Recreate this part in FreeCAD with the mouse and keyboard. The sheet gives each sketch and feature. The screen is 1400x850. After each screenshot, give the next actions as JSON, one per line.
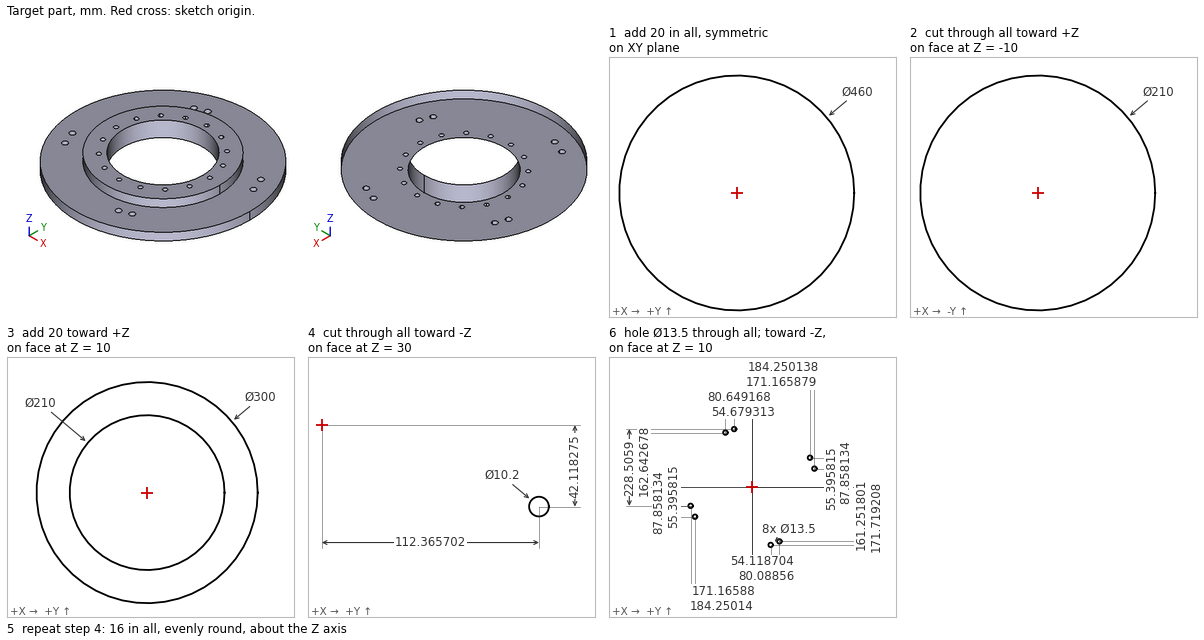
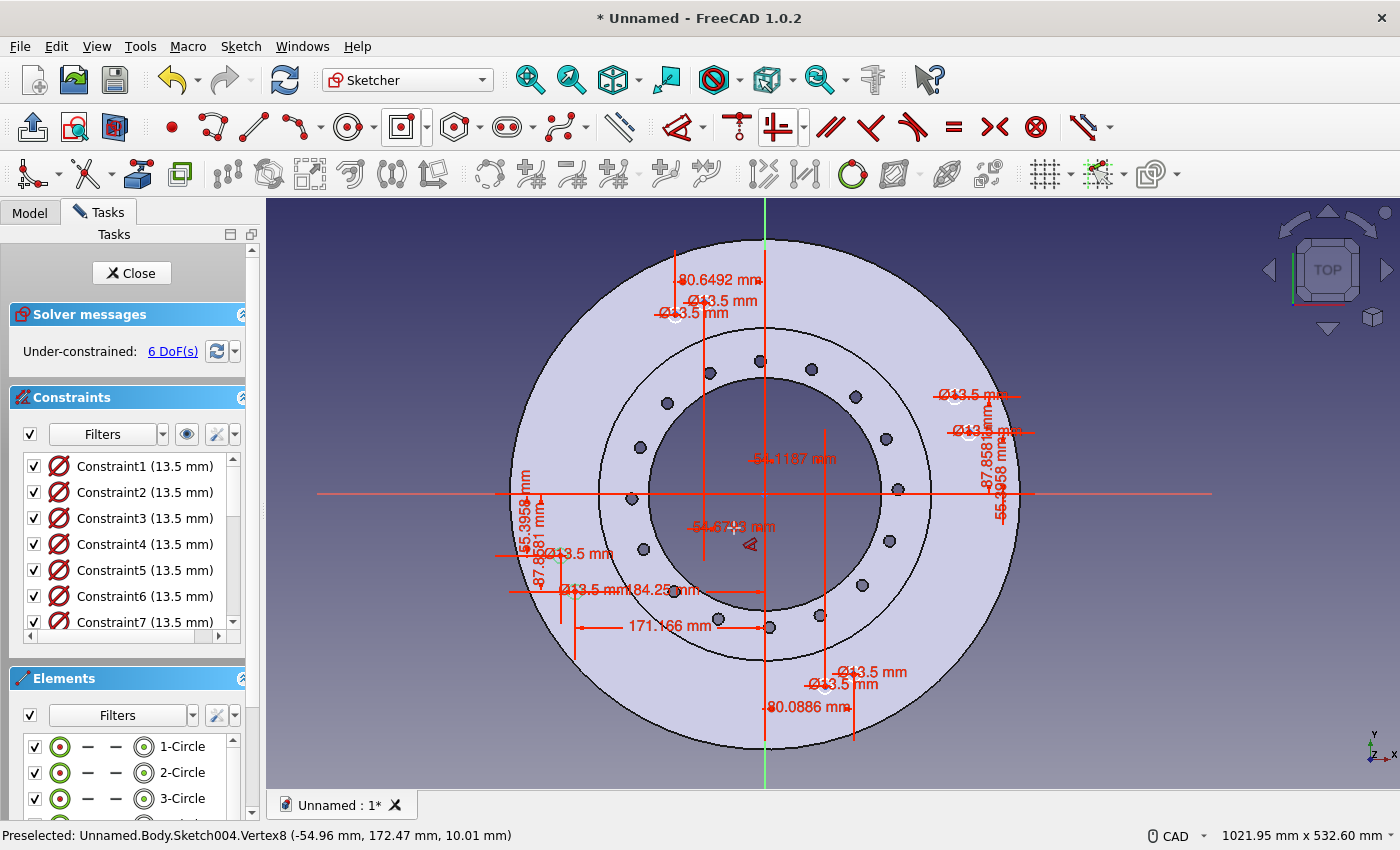
{"action": "left_click", "coordinate": [561, 556]}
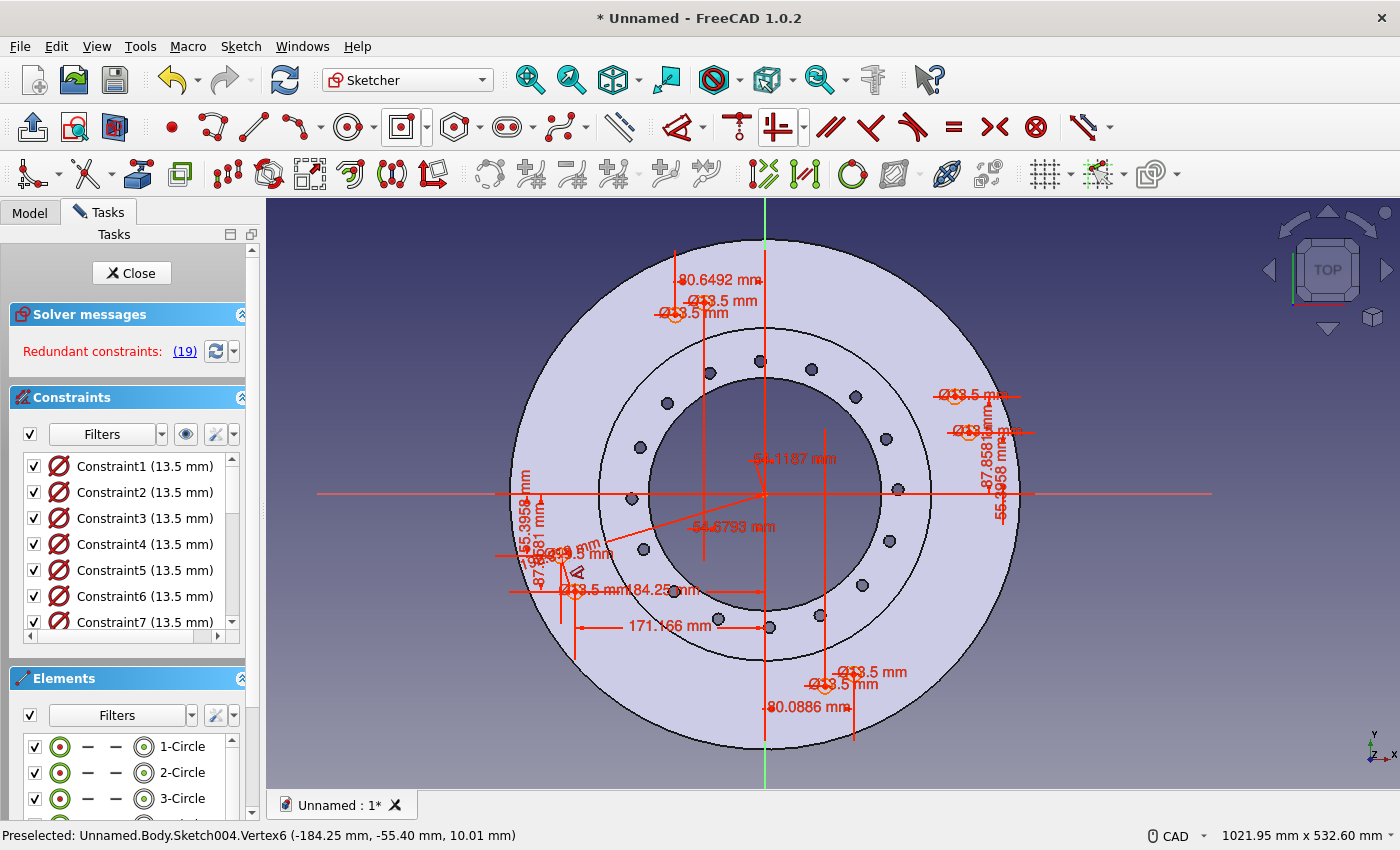
{"action": "left_click", "coordinate": [704, 303]}
{"action": "left_click", "coordinate": [527, 429]}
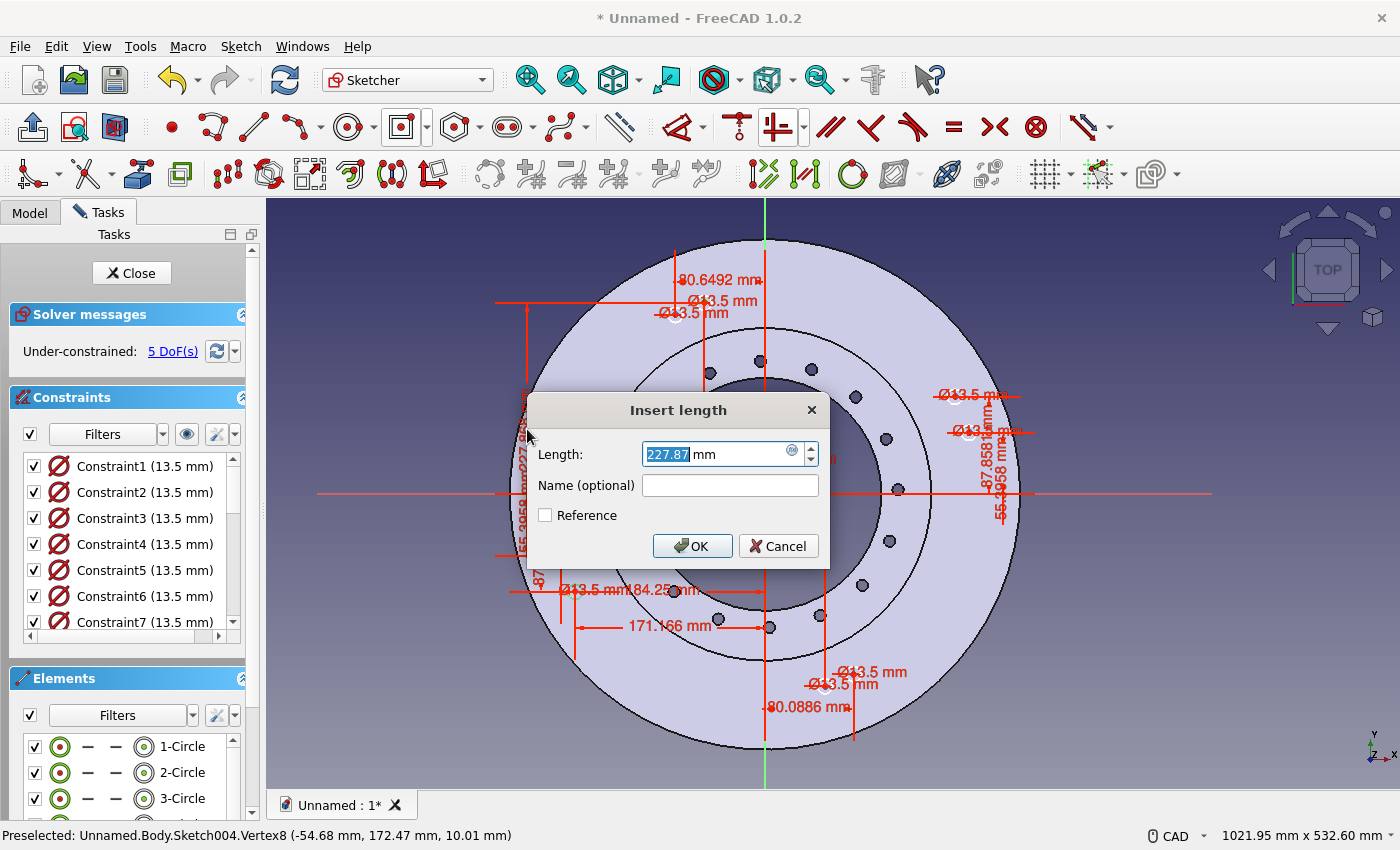
{"action": "type", "text": "228.5059"}
{"action": "key", "text": "Return"}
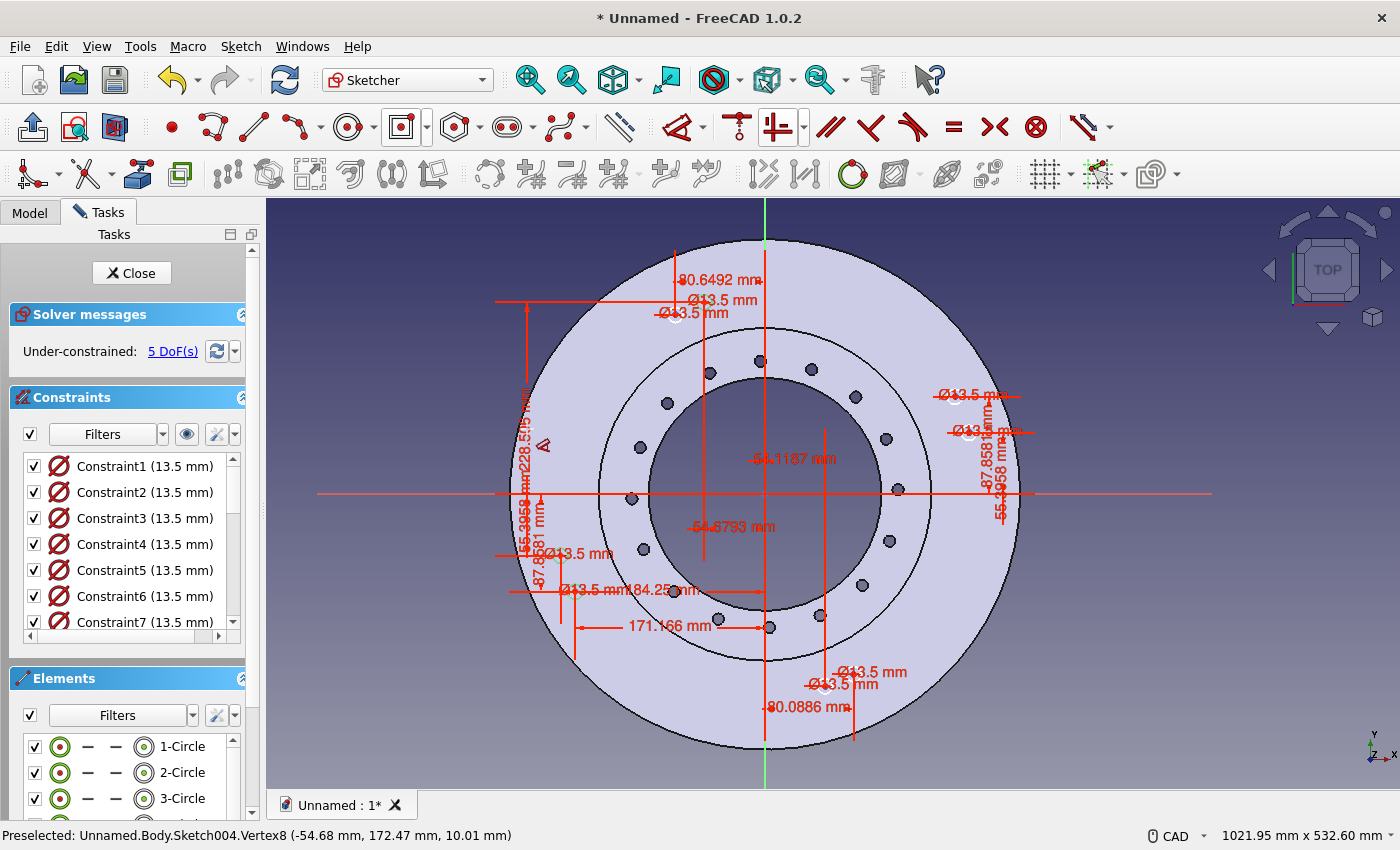
{"action": "left_click", "coordinate": [825, 686]}
{"action": "left_click", "coordinate": [859, 590]}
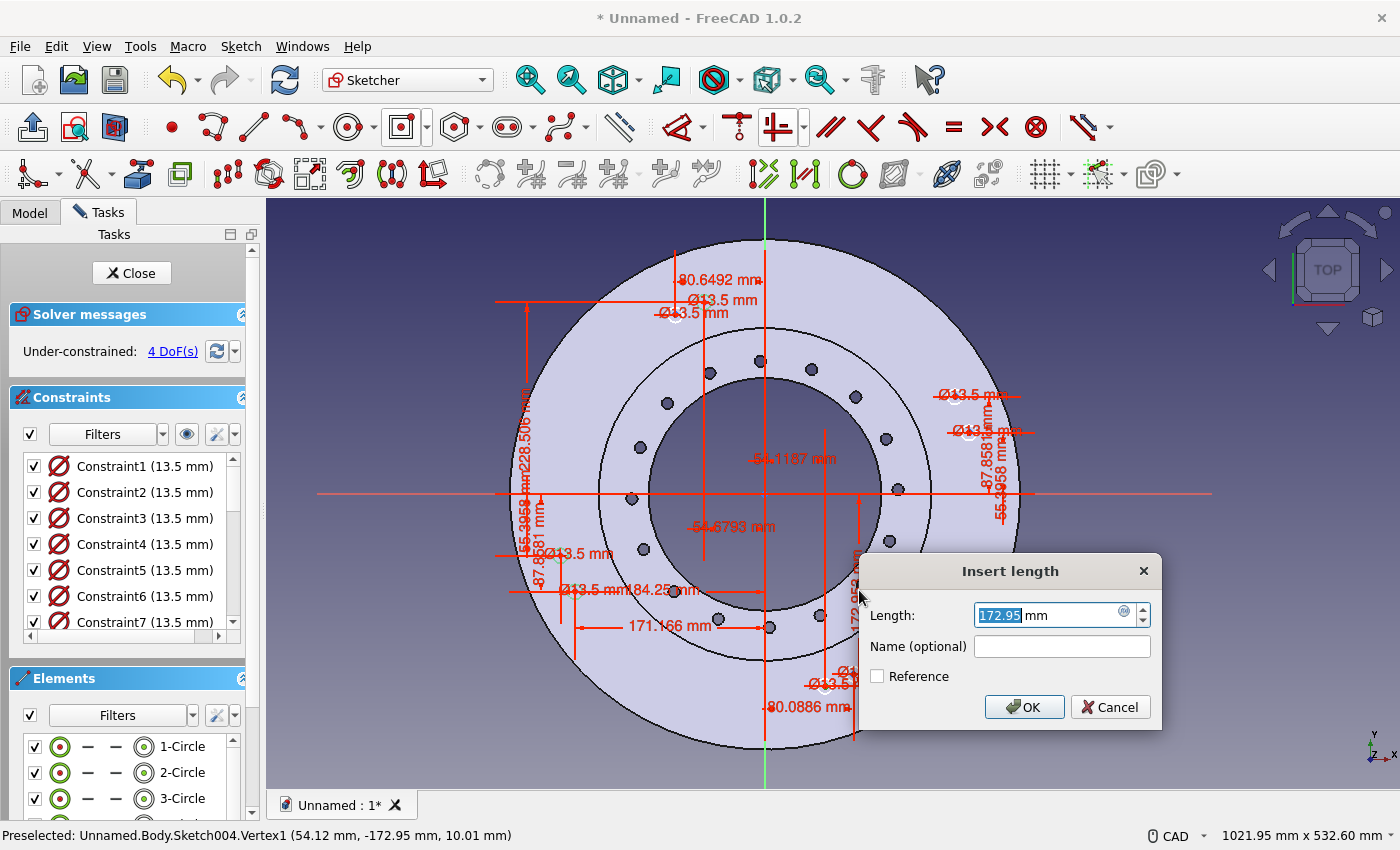
{"action": "type", "text": "171.719208"}
{"action": "key", "text": "Return"}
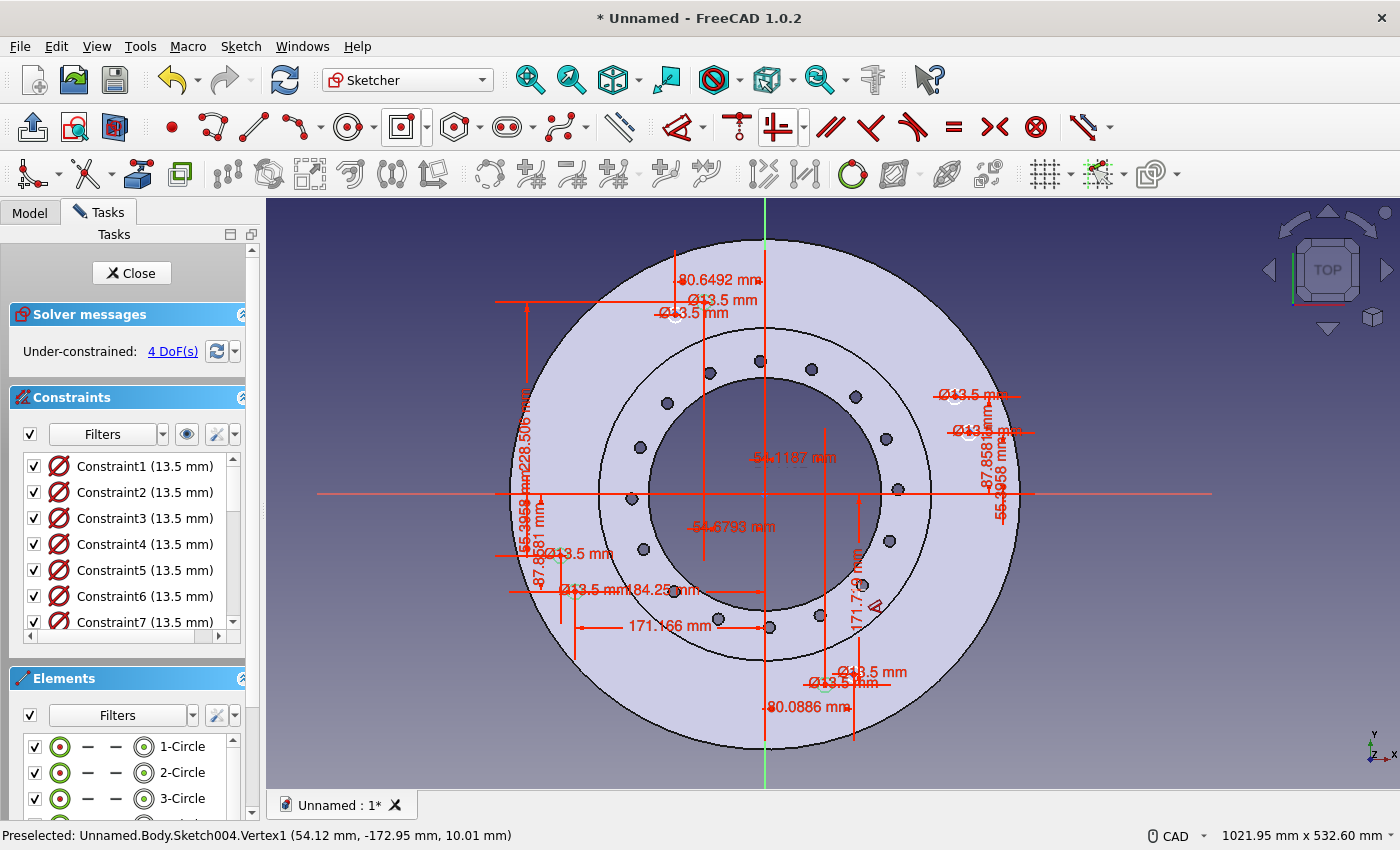
{"action": "left_click", "coordinate": [854, 674]}
{"action": "left_click", "coordinate": [888, 543]}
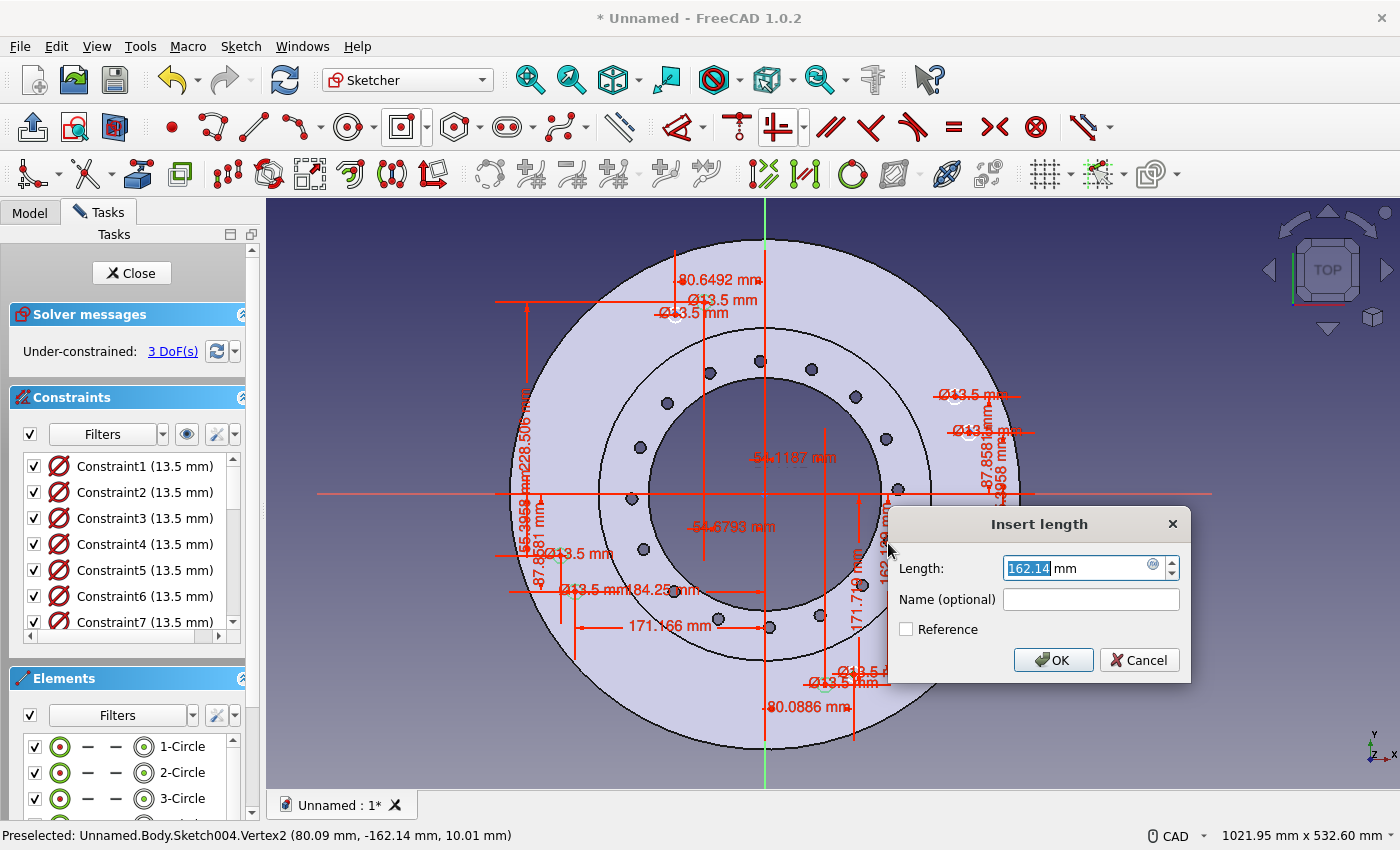
{"action": "type", "text": "161.251801"}
{"action": "key", "text": "Return"}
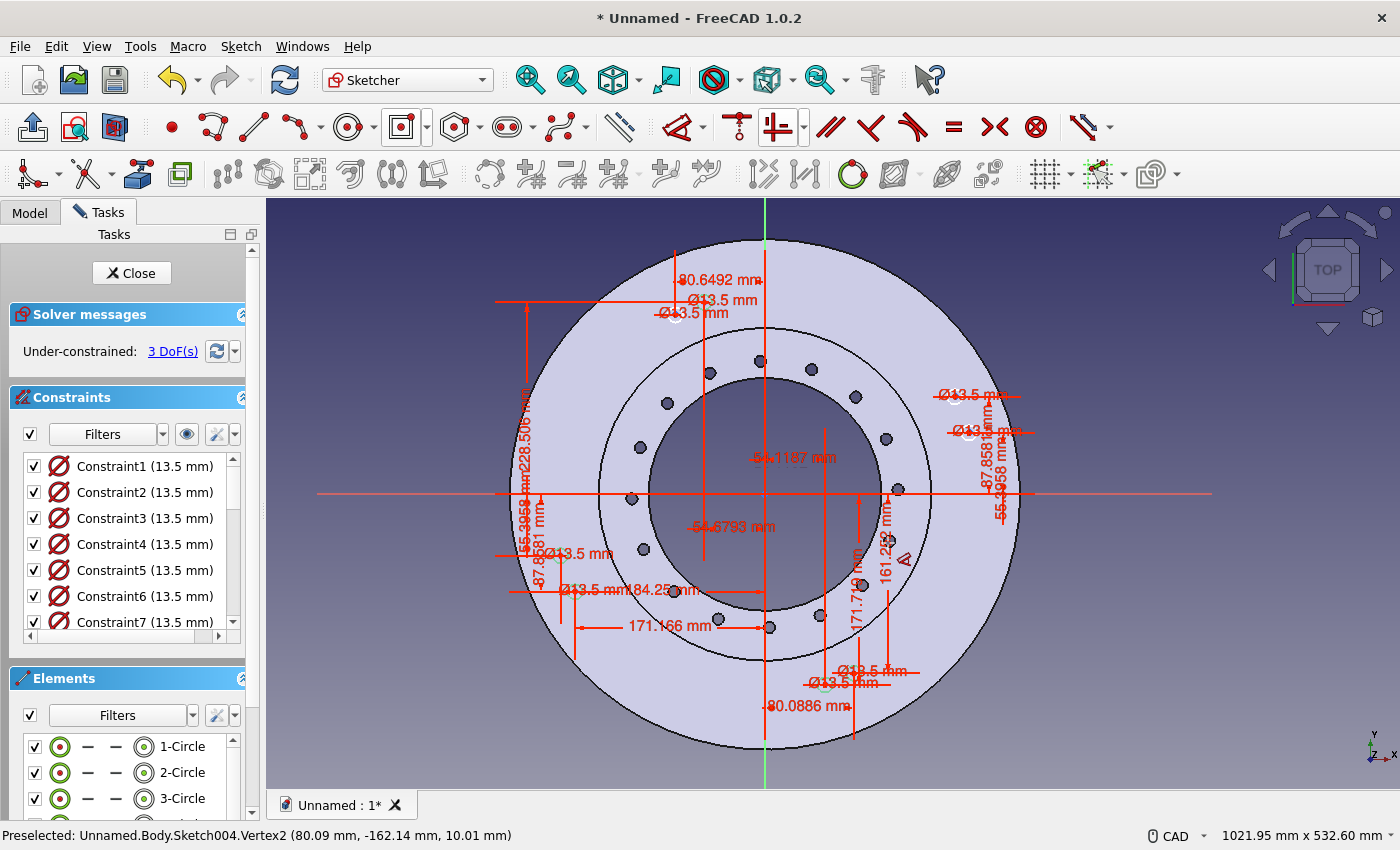
{"action": "left_click", "coordinate": [955, 397]}
{"action": "left_click", "coordinate": [860, 363]}